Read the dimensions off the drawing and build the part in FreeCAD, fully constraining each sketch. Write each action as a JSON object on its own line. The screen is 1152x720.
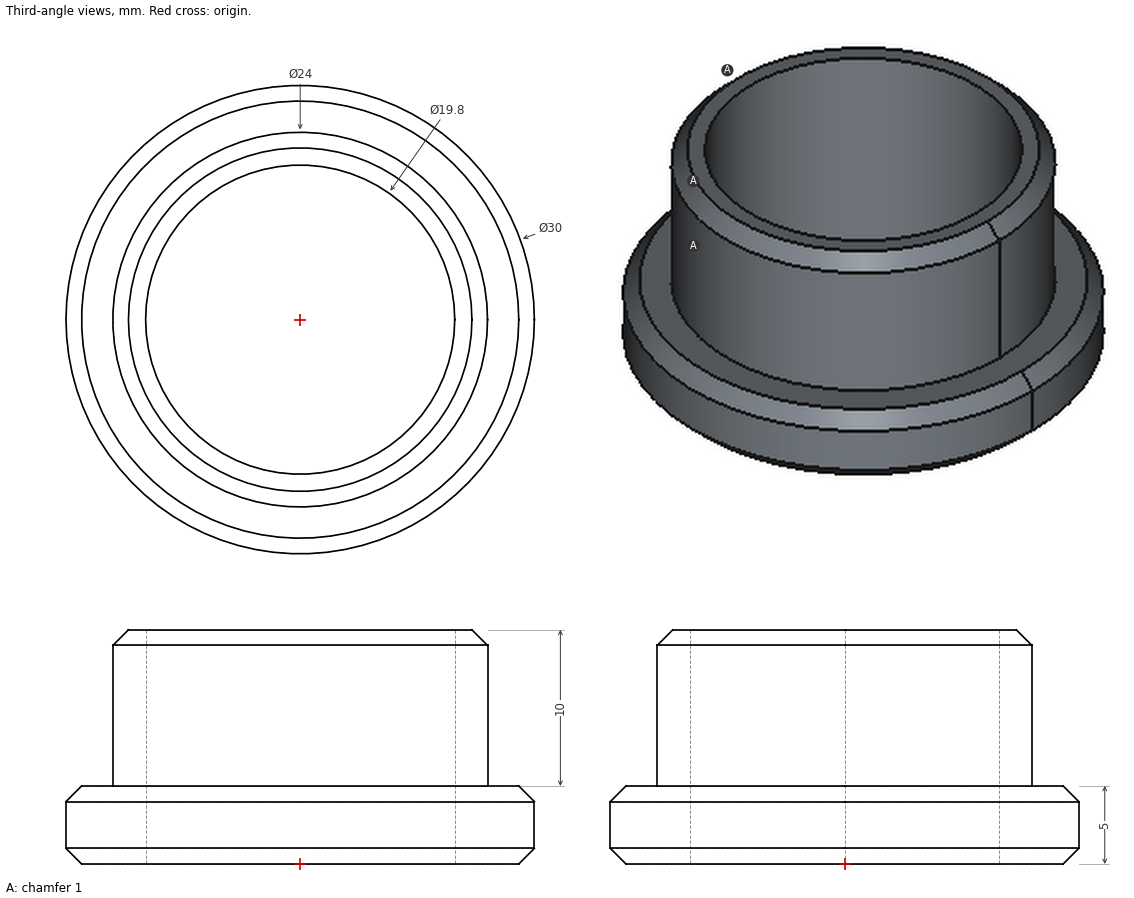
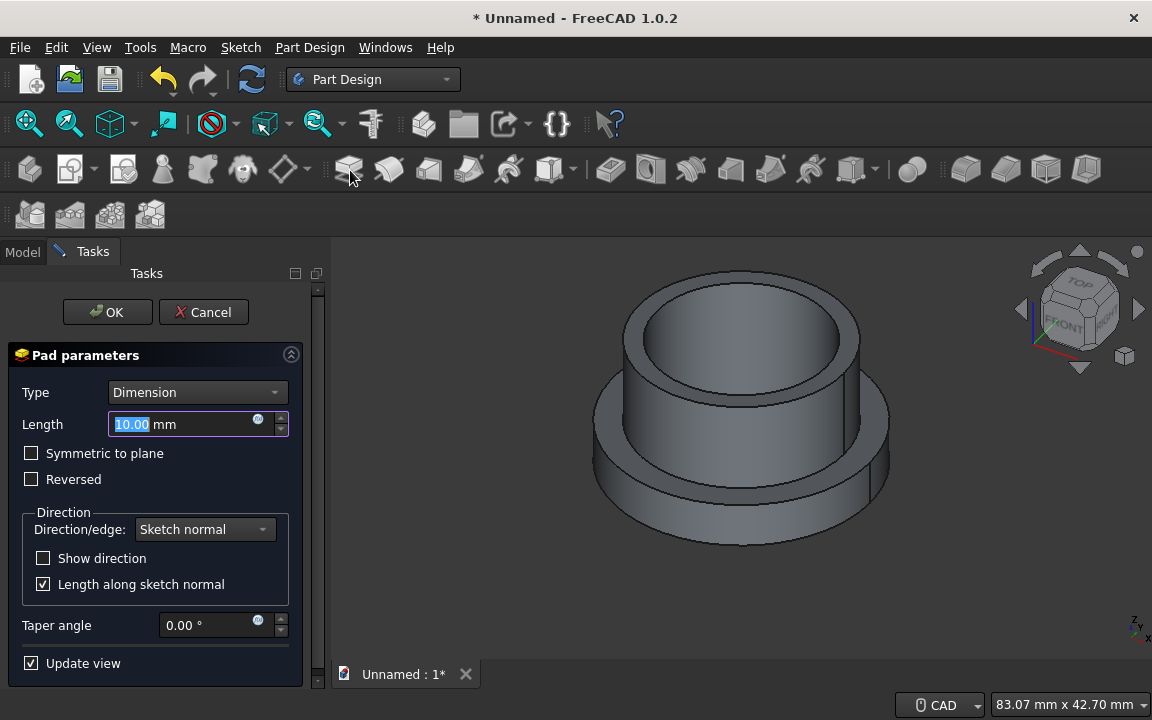
{"action": "type", "text": "10"}
{"action": "key", "text": "Tab"}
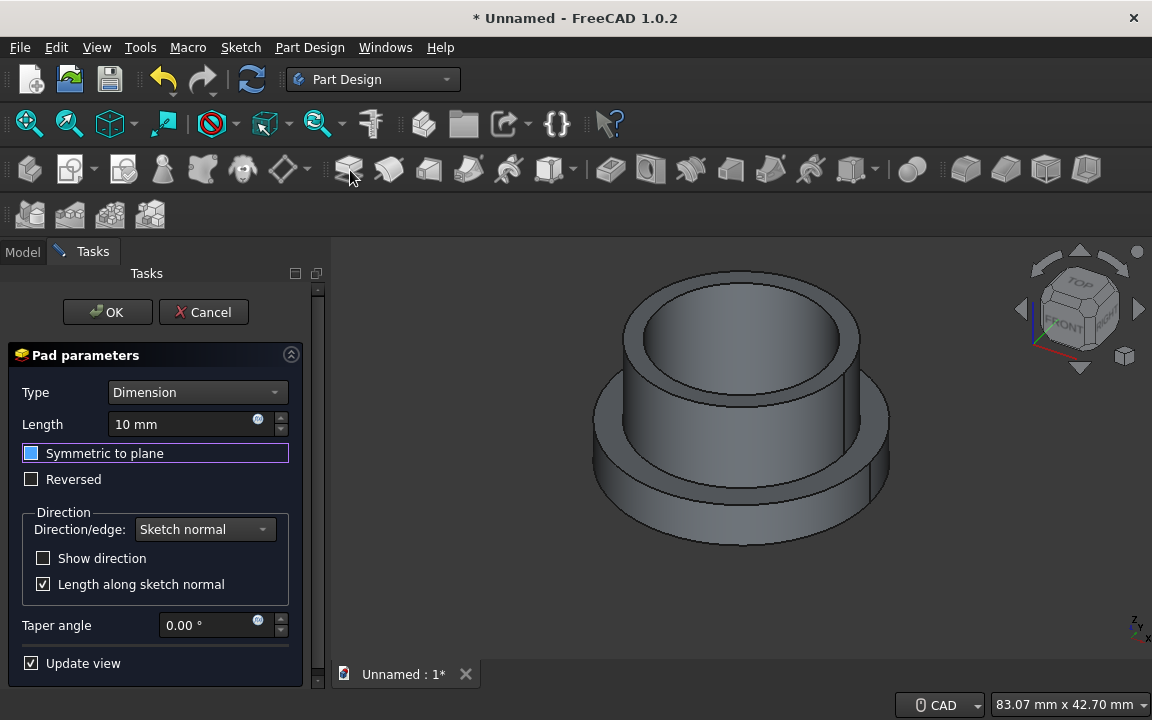
{"action": "left_click", "coordinate": [108, 312]}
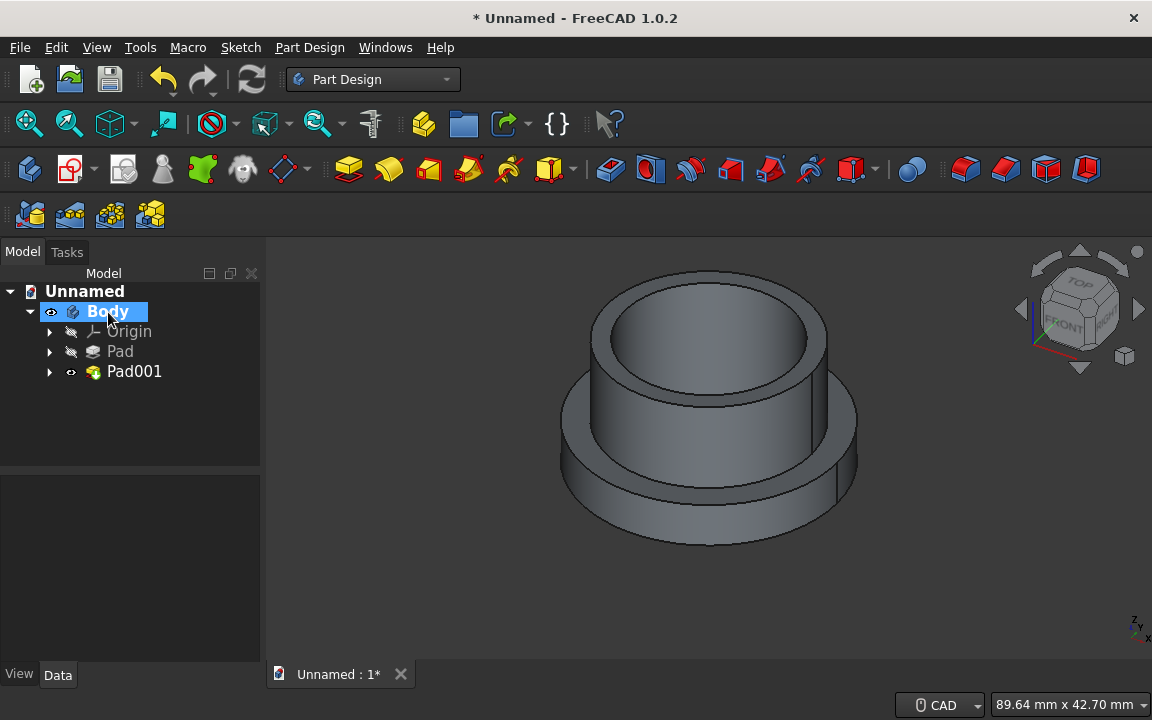
{"action": "left_click", "coordinate": [30, 124]}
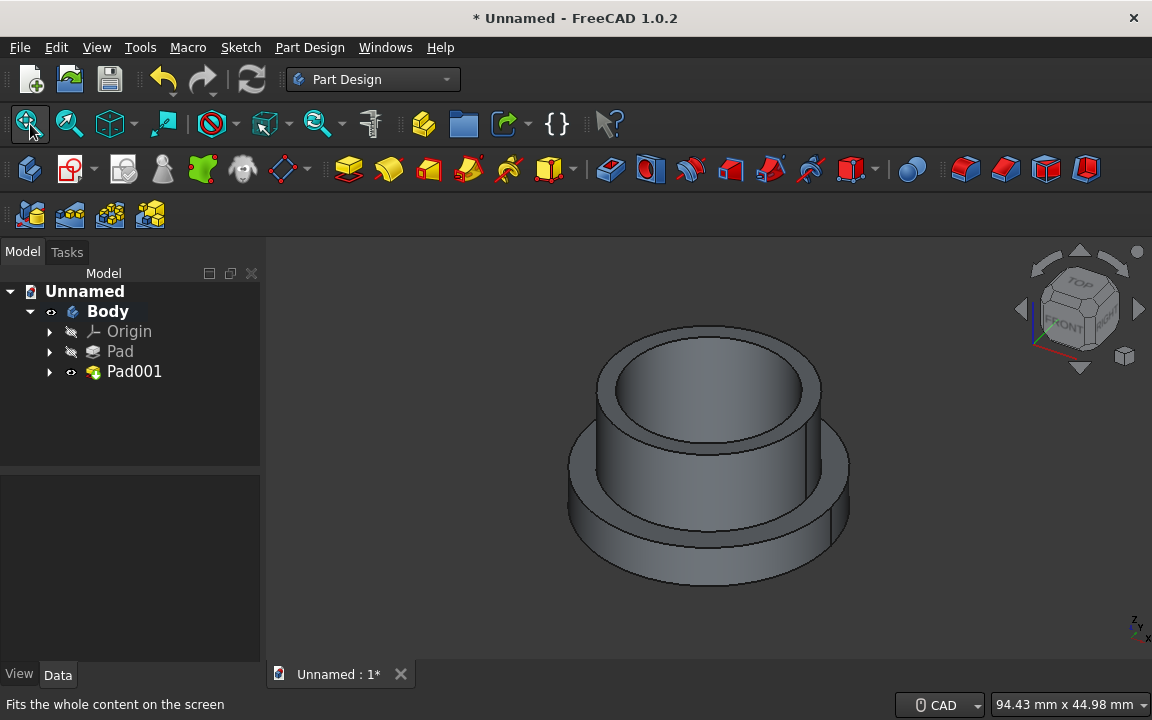
{"action": "left_click", "coordinate": [597, 396]}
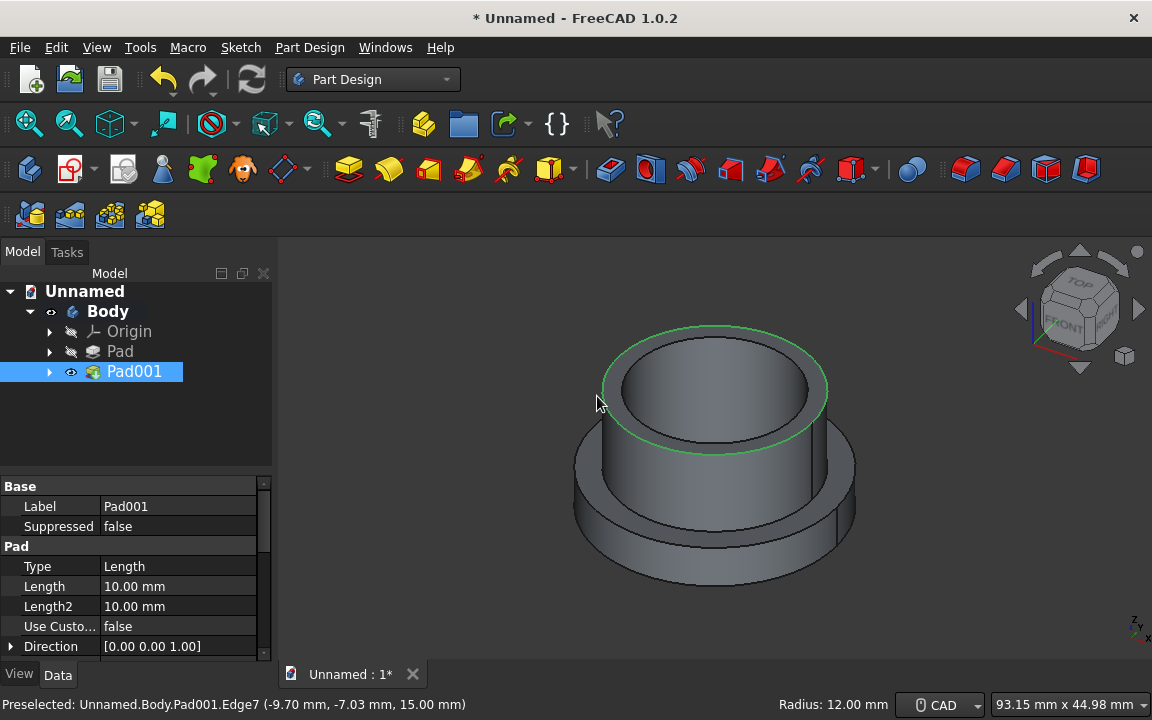
{"action": "left_click", "coordinate": [575, 475], "text": "ctrl"}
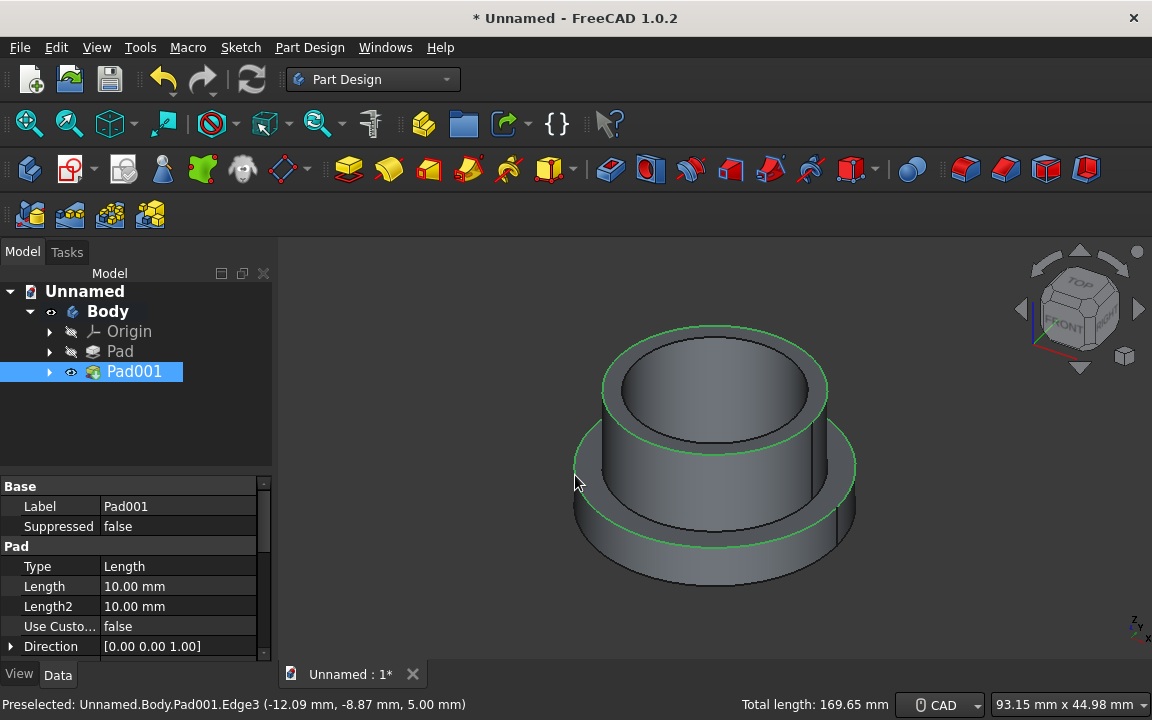
{"action": "key", "text": "0"}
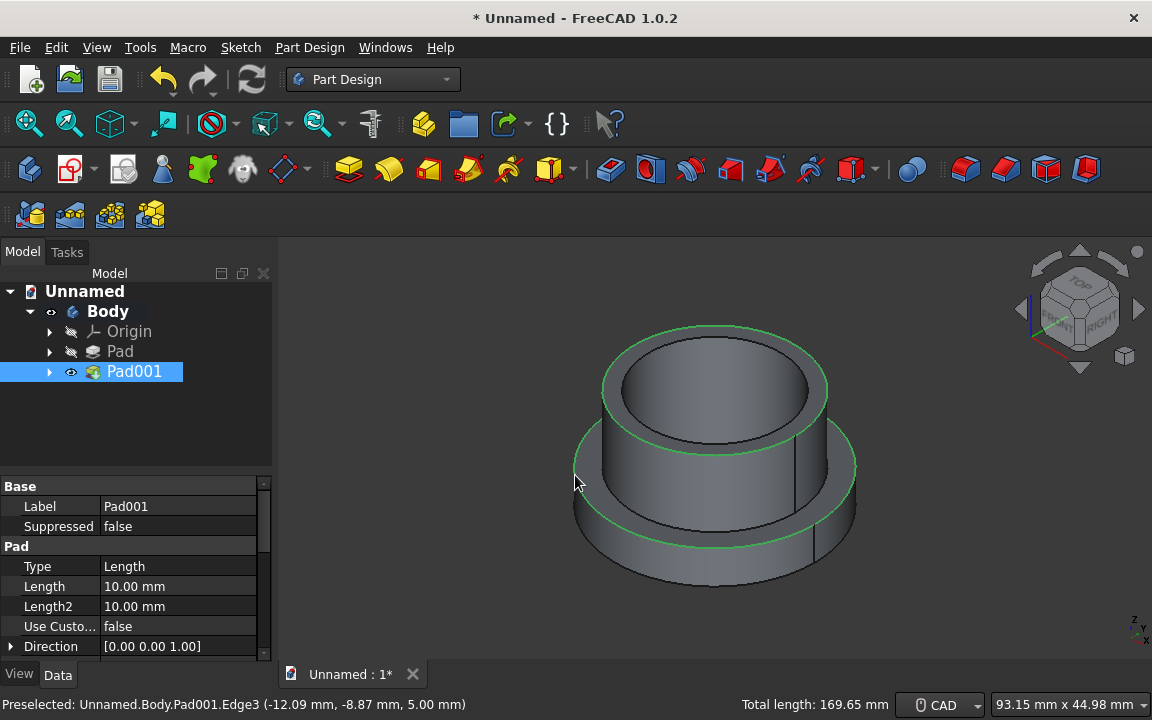
{"action": "key", "text": "2"}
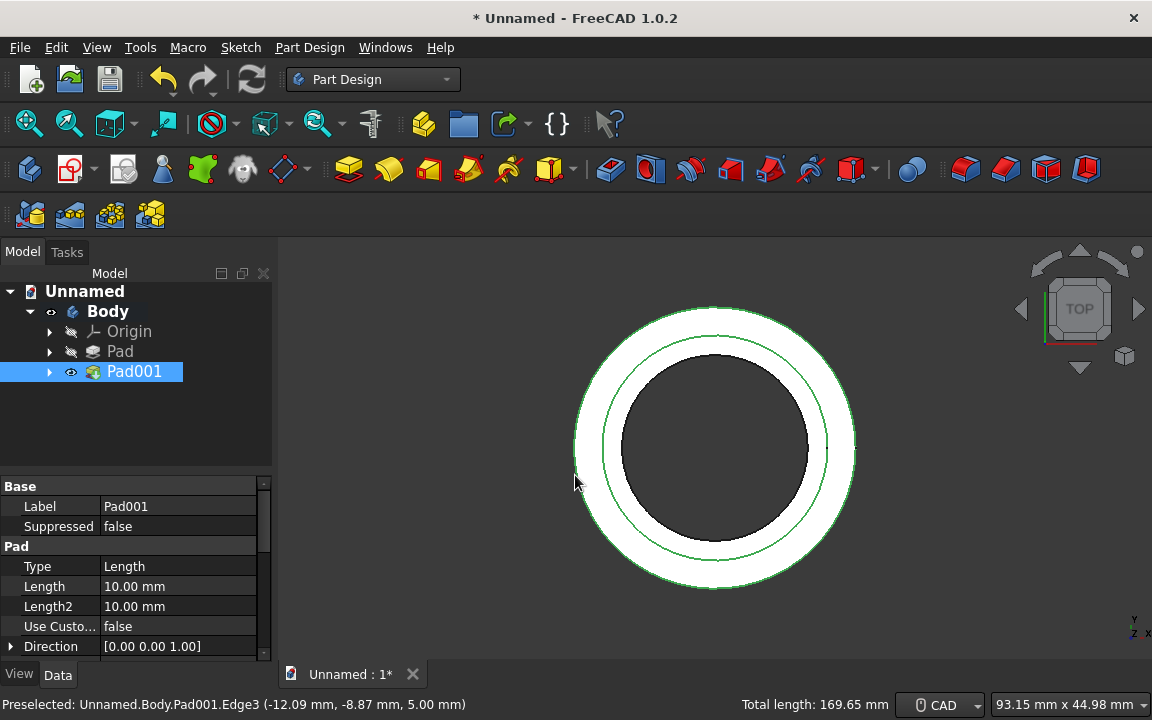
{"action": "key", "text": "1"}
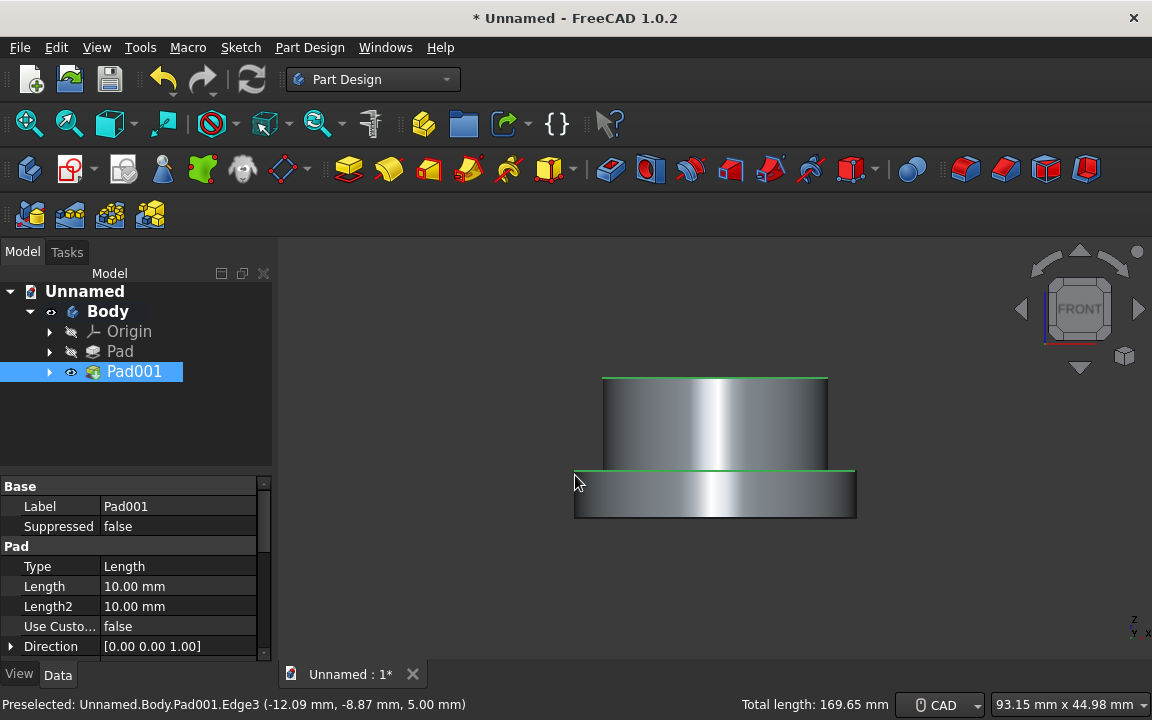
{"action": "left_click", "coordinate": [30, 124]}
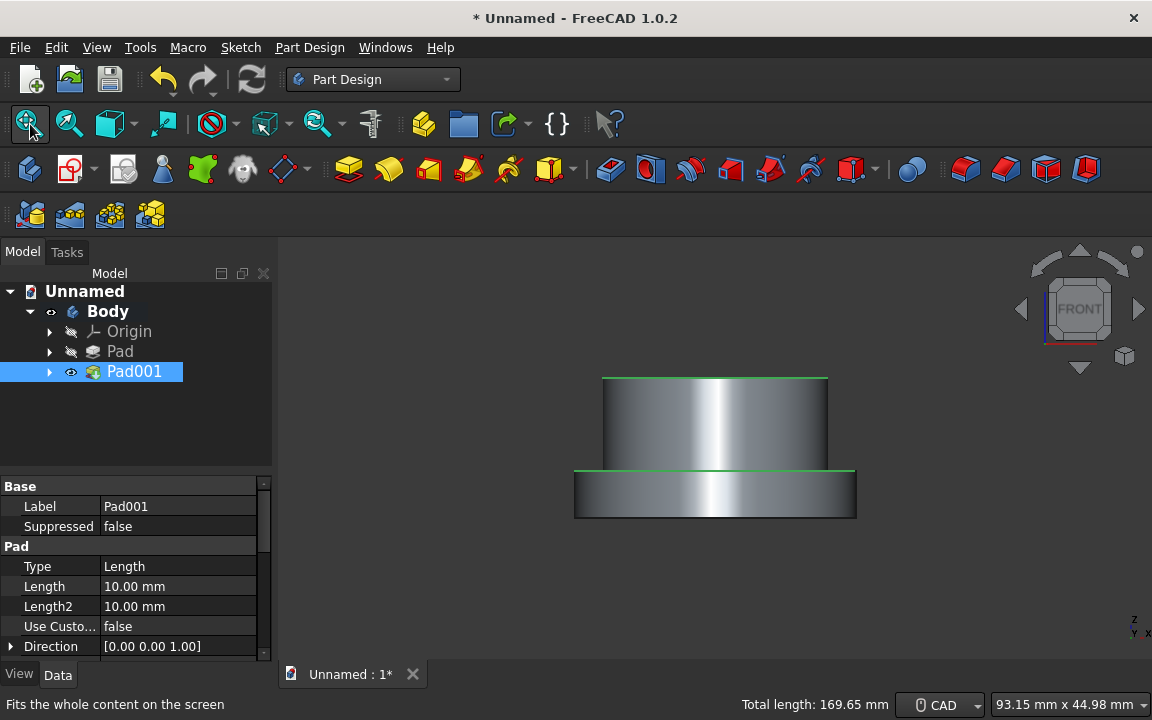
{"action": "left_click", "coordinate": [601, 517], "text": "ctrl"}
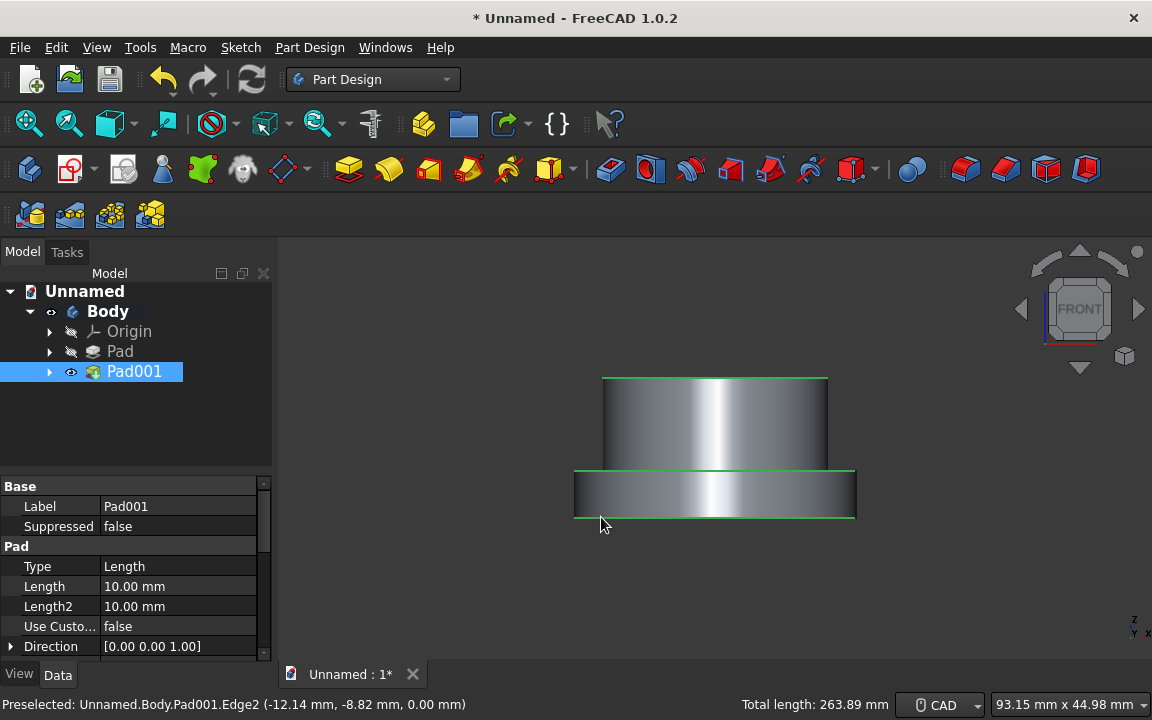
{"action": "left_click", "coordinate": [1006, 170]}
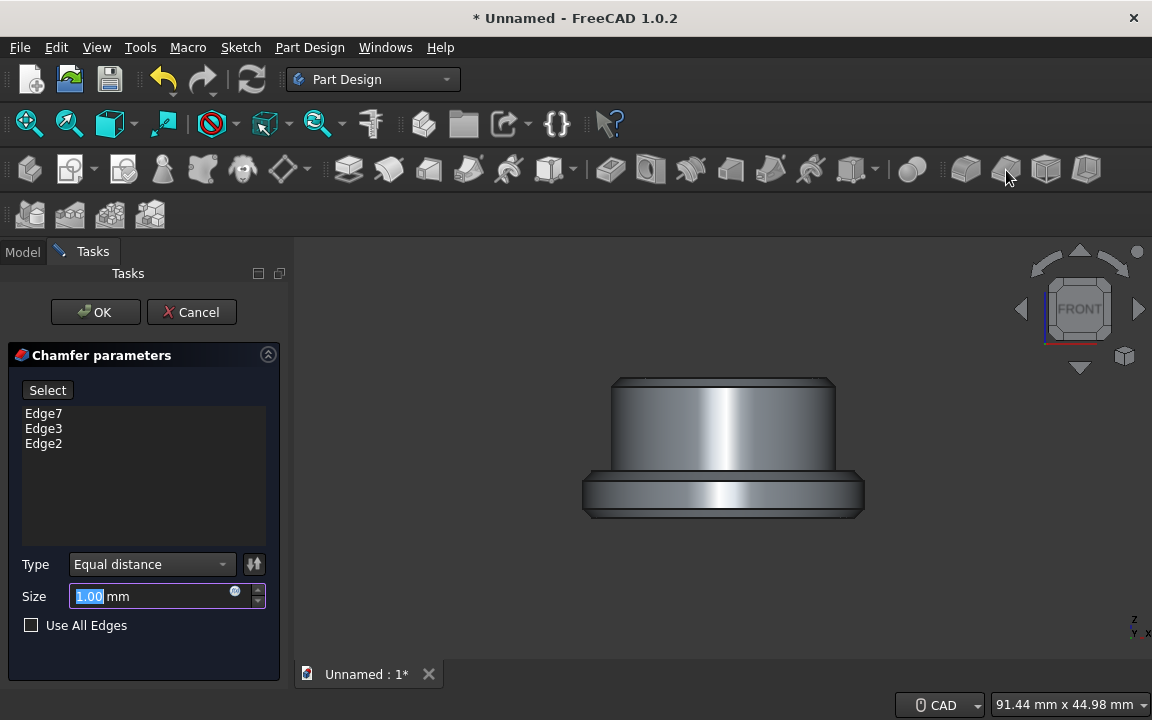
{"action": "type", "text": "1"}
{"action": "key", "text": "Tab"}